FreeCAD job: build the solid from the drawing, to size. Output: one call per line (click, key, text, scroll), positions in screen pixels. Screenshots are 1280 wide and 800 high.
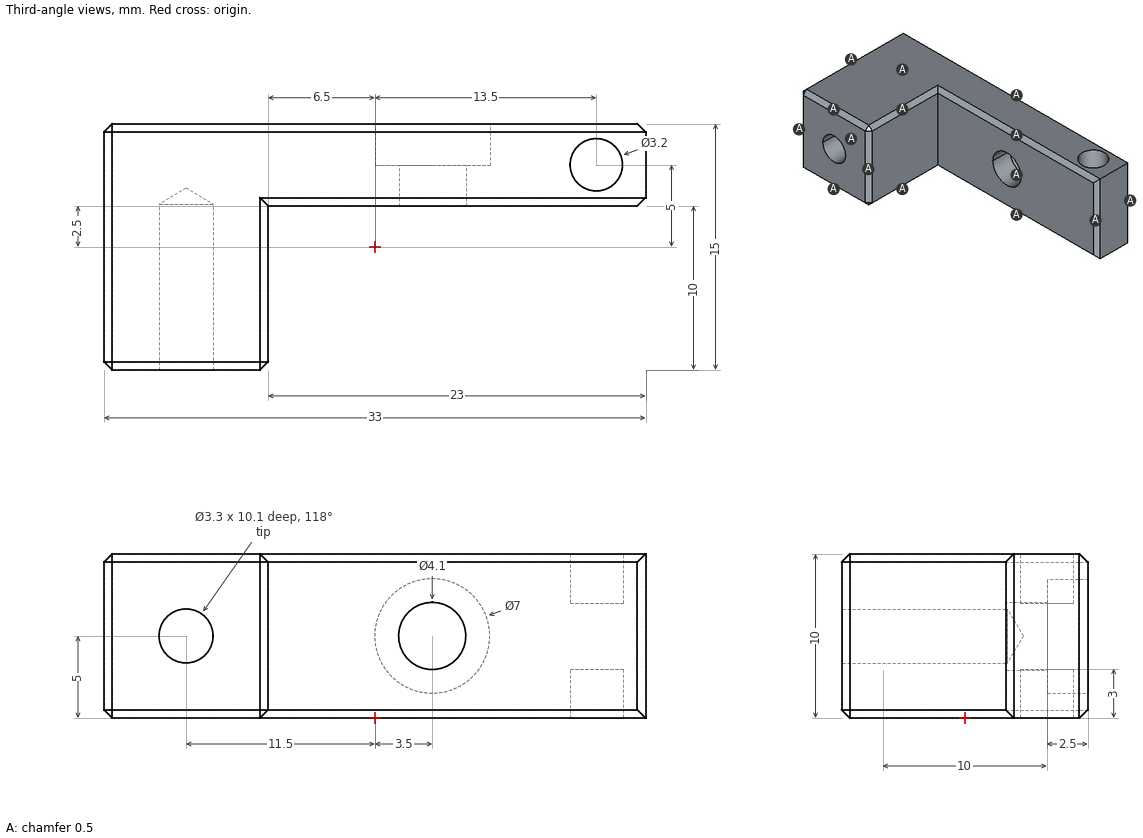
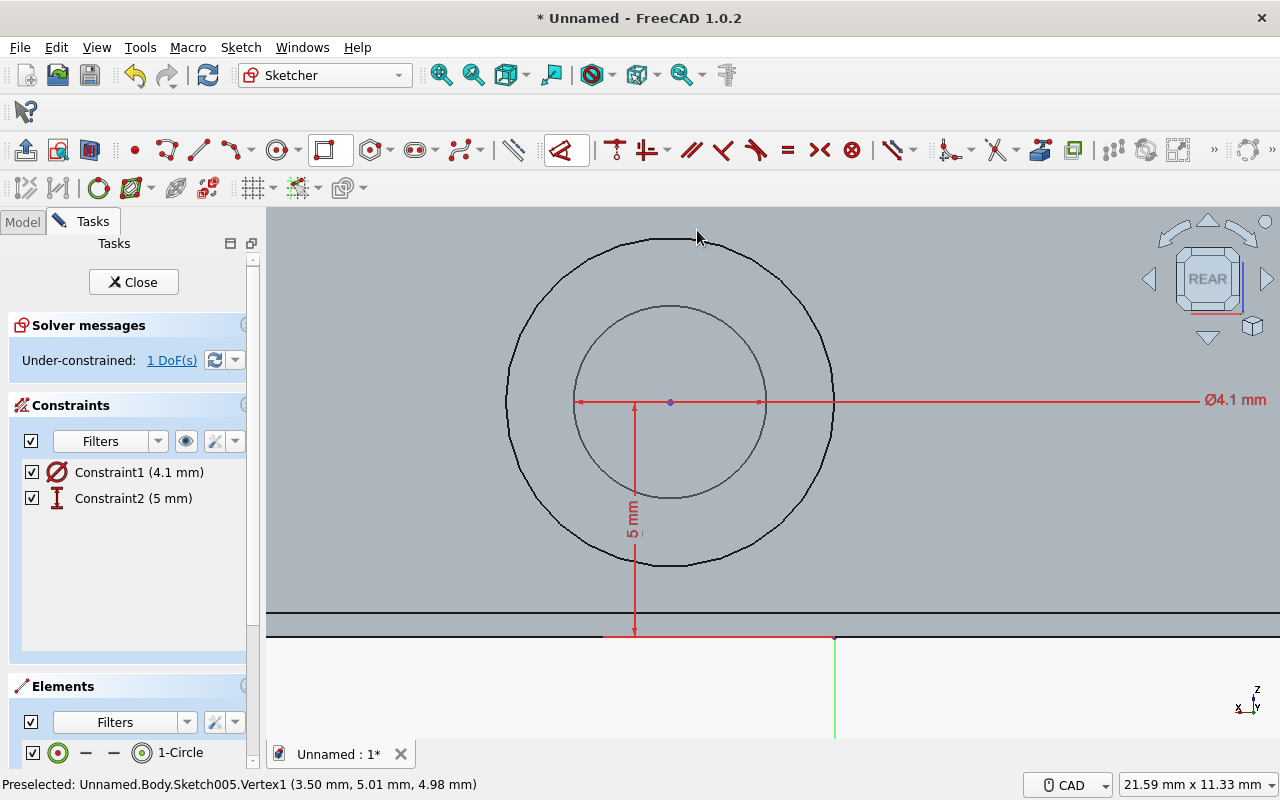
click(670, 402)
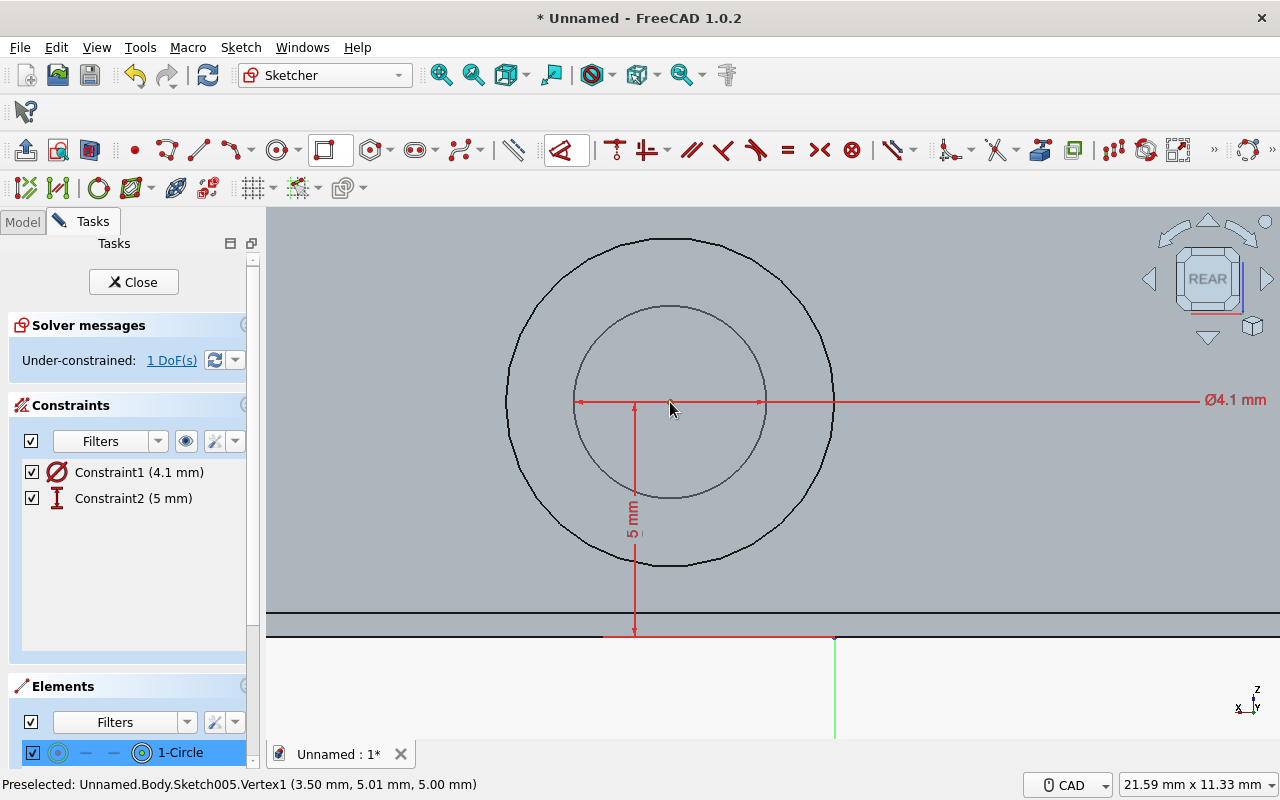
key(l)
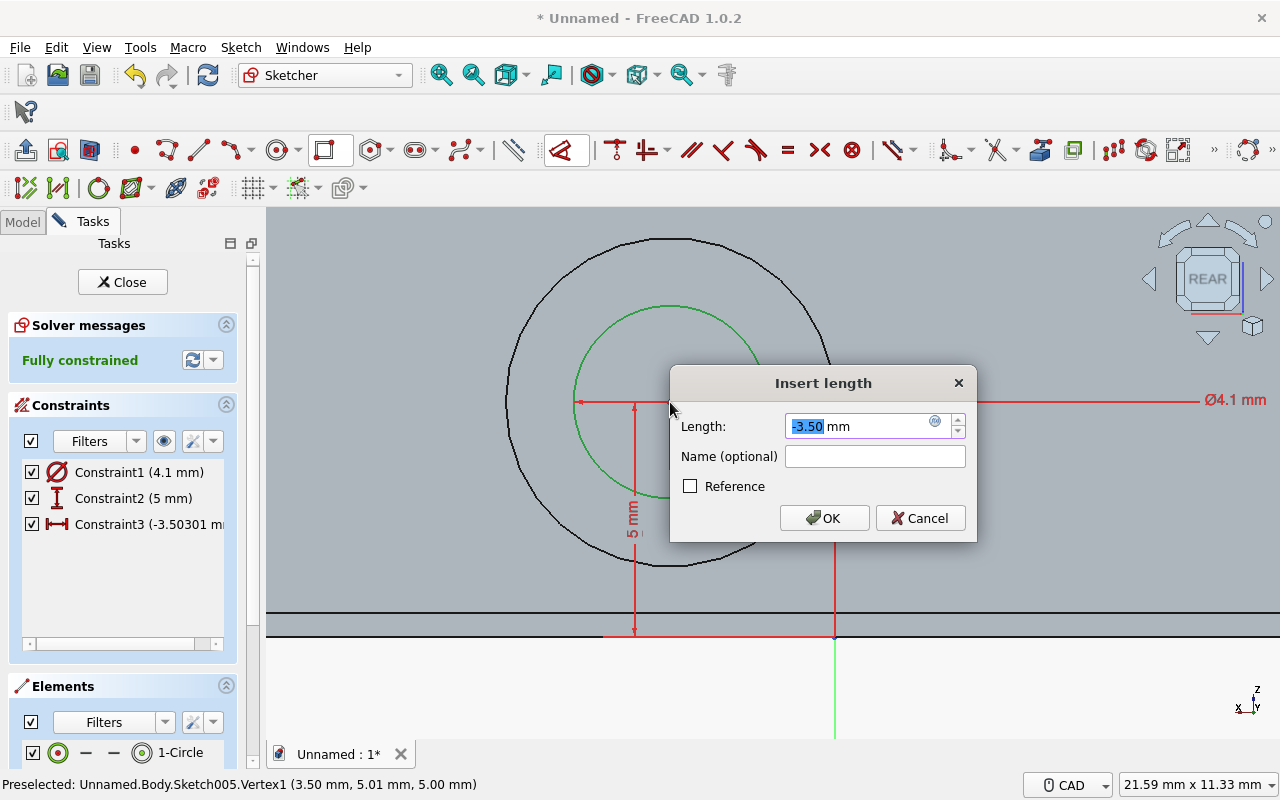
text(-3.5)
key(Return)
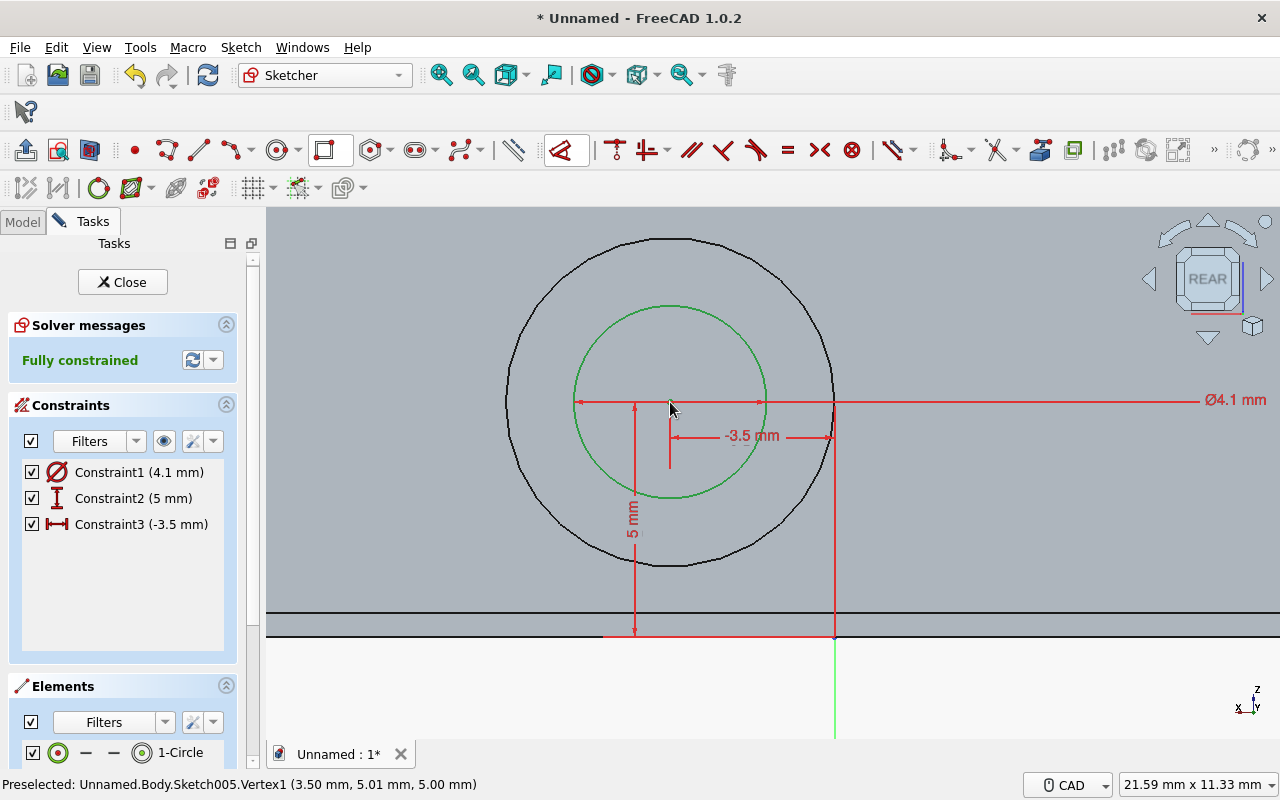
click(123, 282)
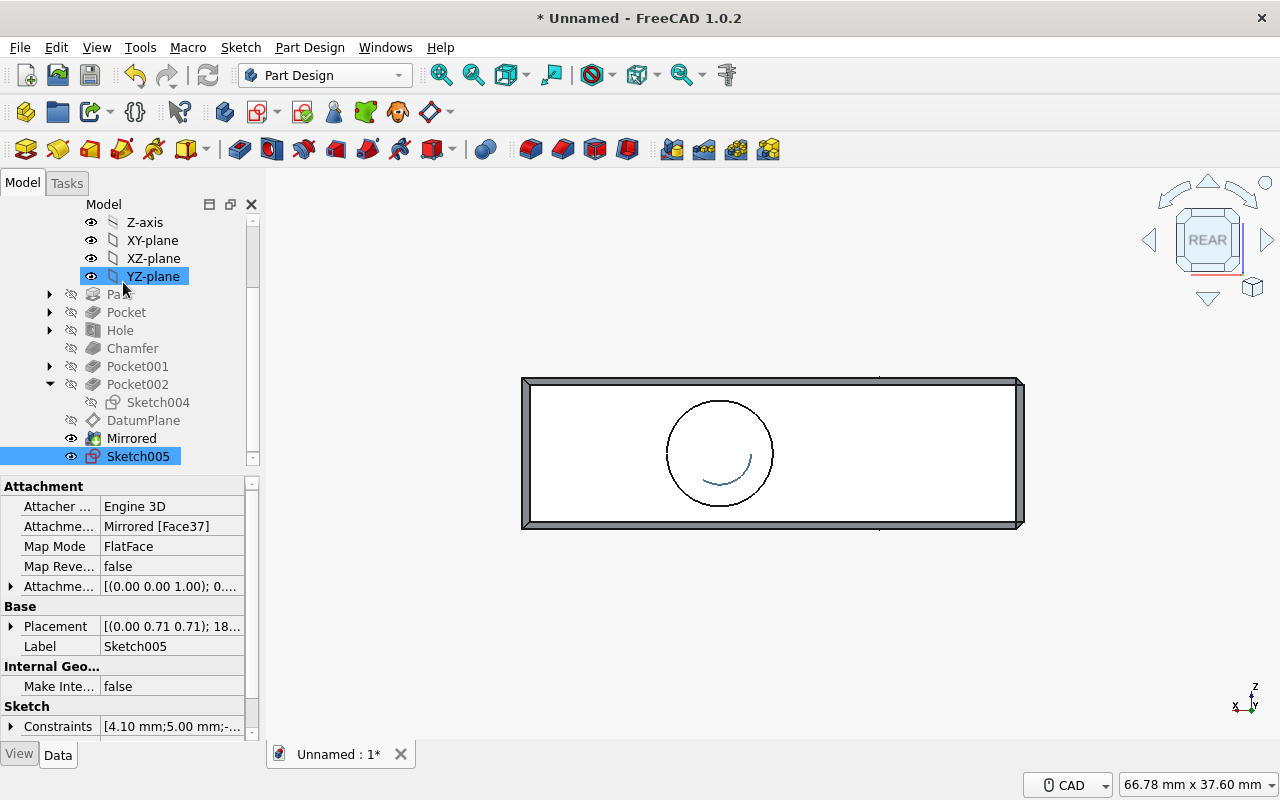
click(240, 150)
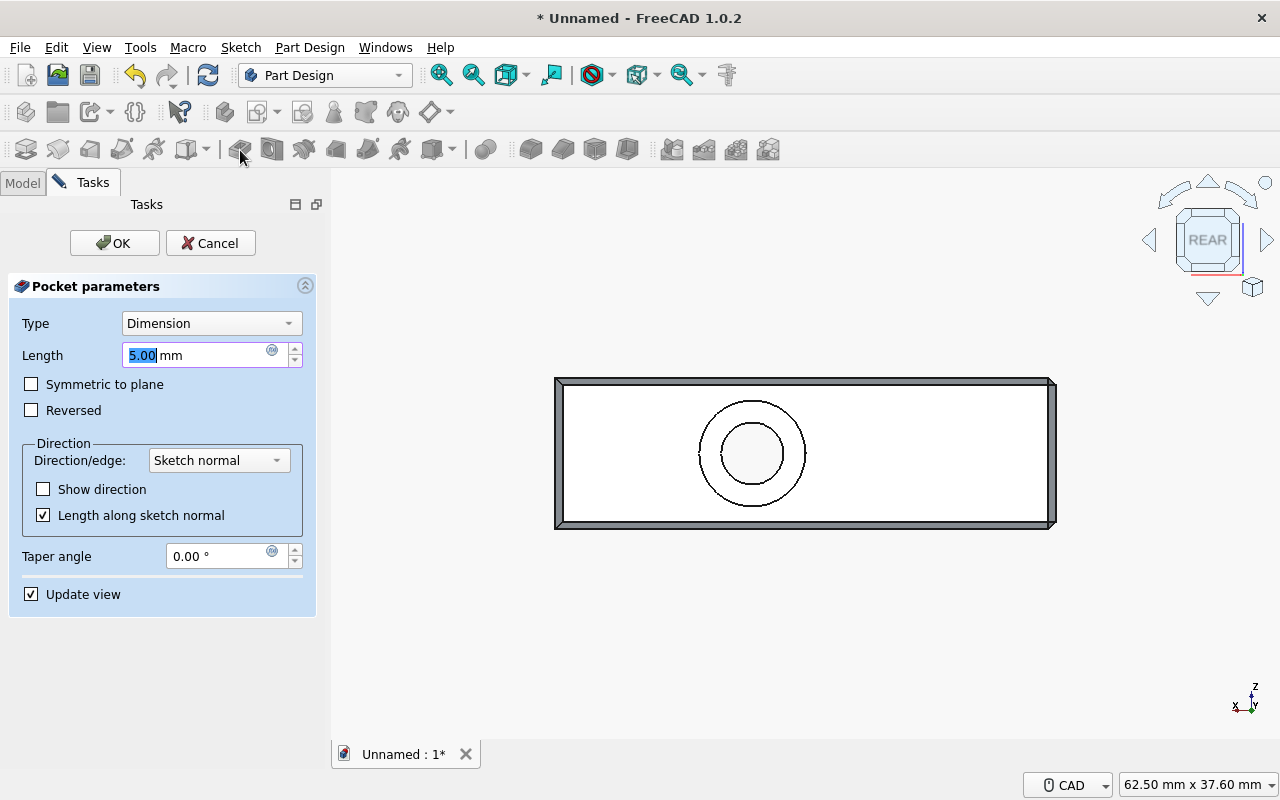
text(10)
key(Tab)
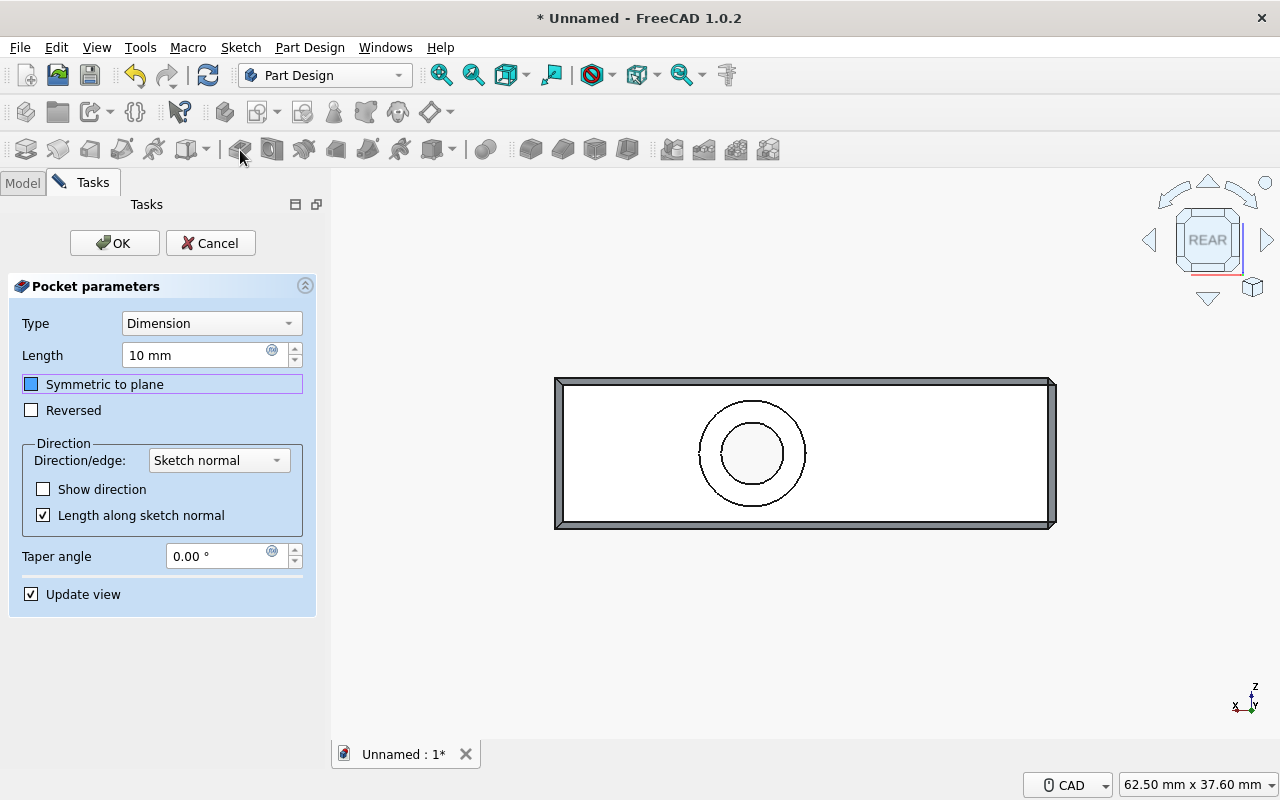
click(115, 243)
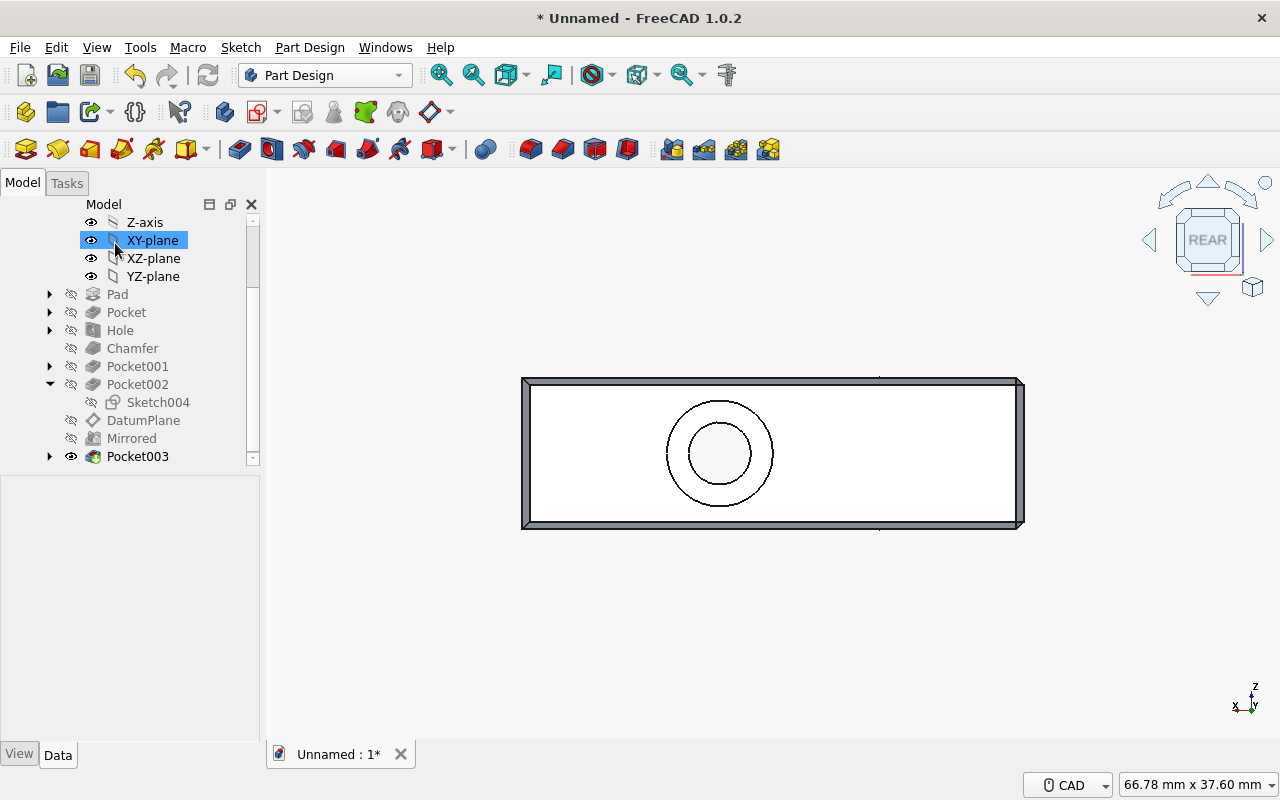
key(0)